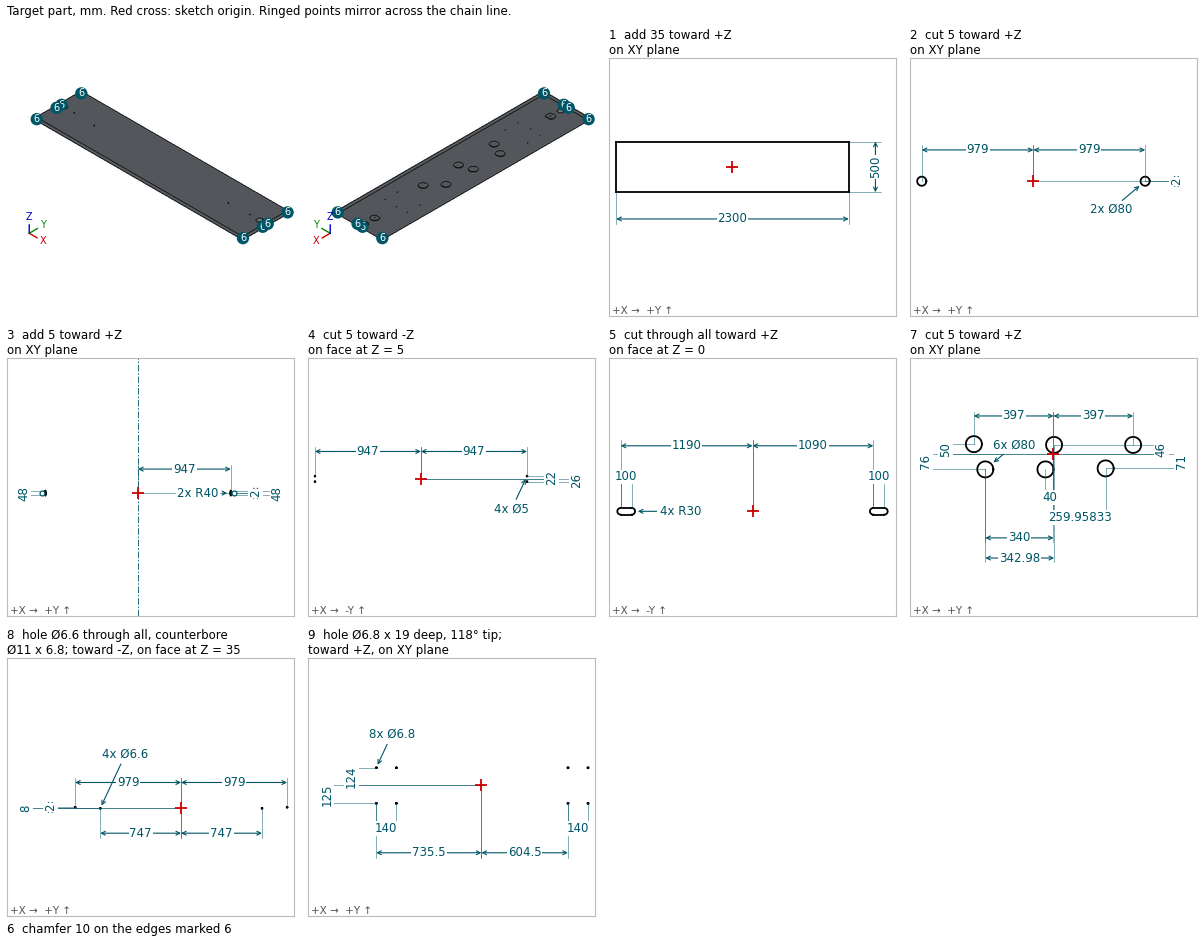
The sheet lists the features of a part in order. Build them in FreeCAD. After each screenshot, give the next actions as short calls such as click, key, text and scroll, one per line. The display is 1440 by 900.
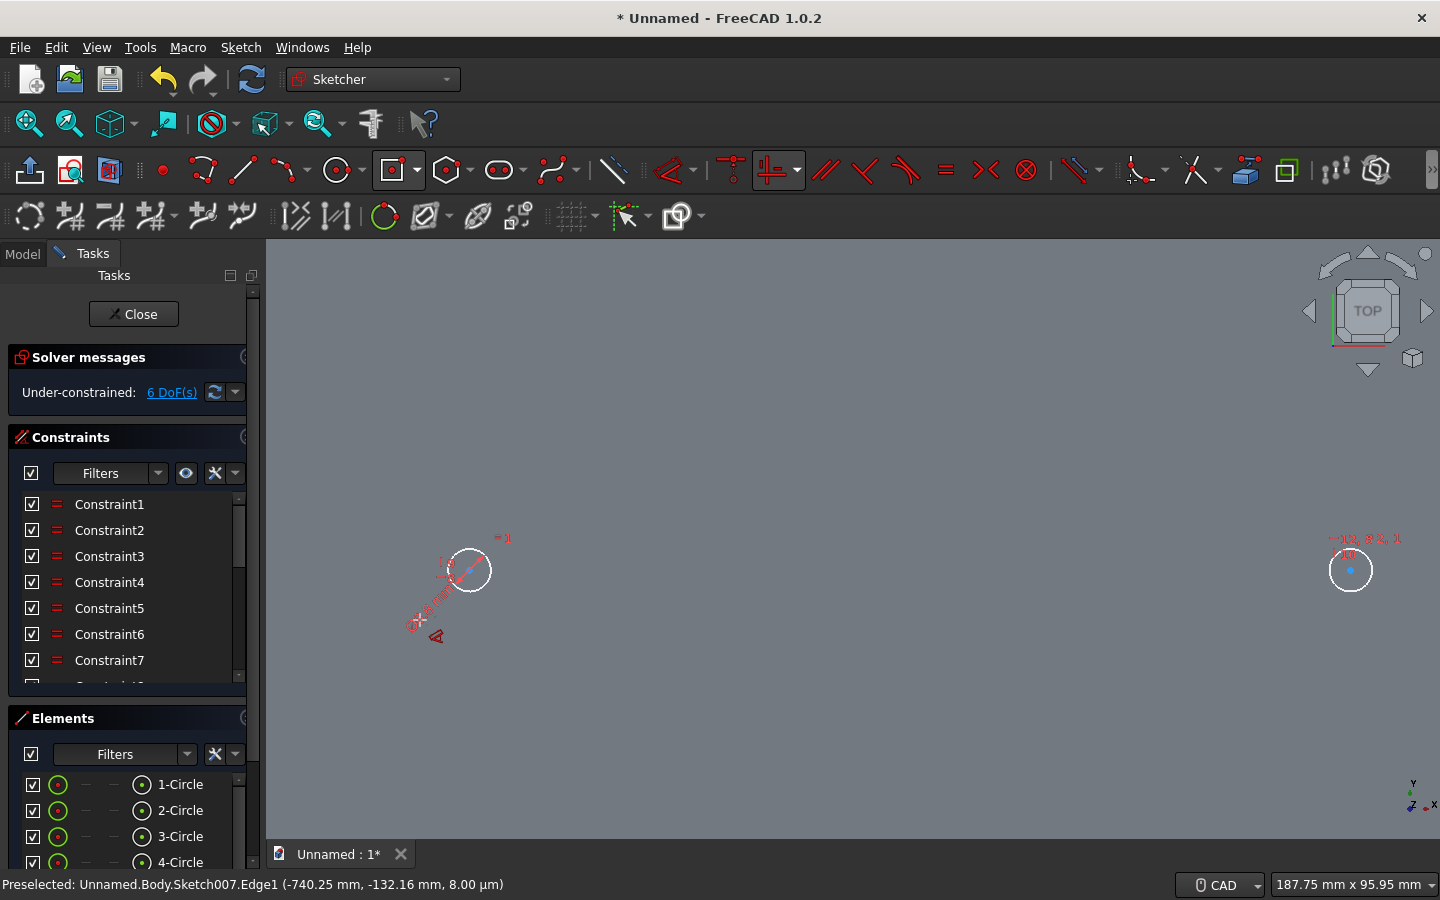
scroll(438, 600, down, 13)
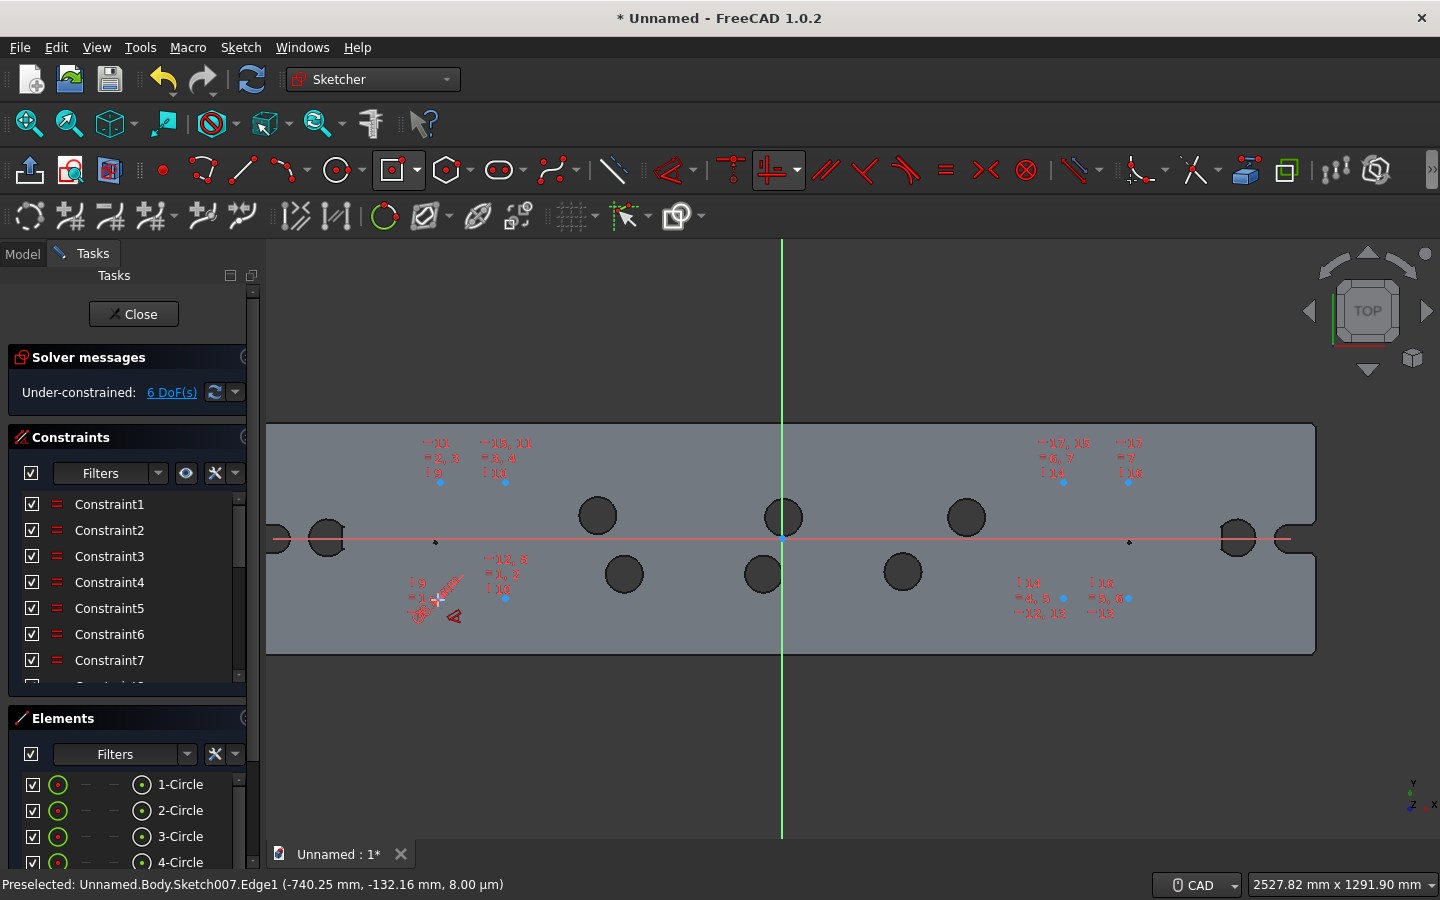
click(440, 598)
click(406, 569)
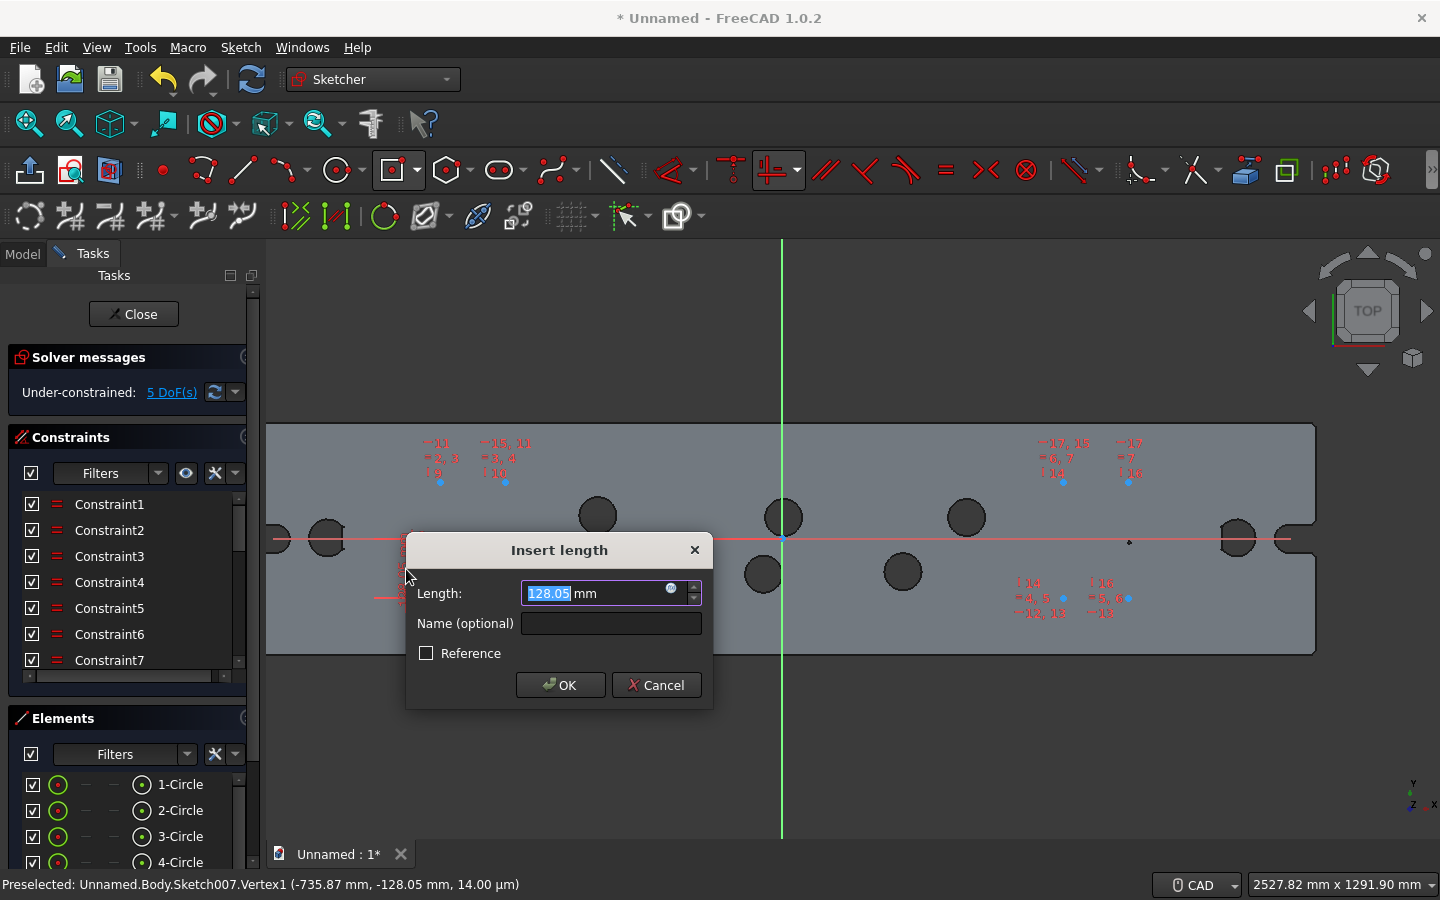
text(125)
key(Return)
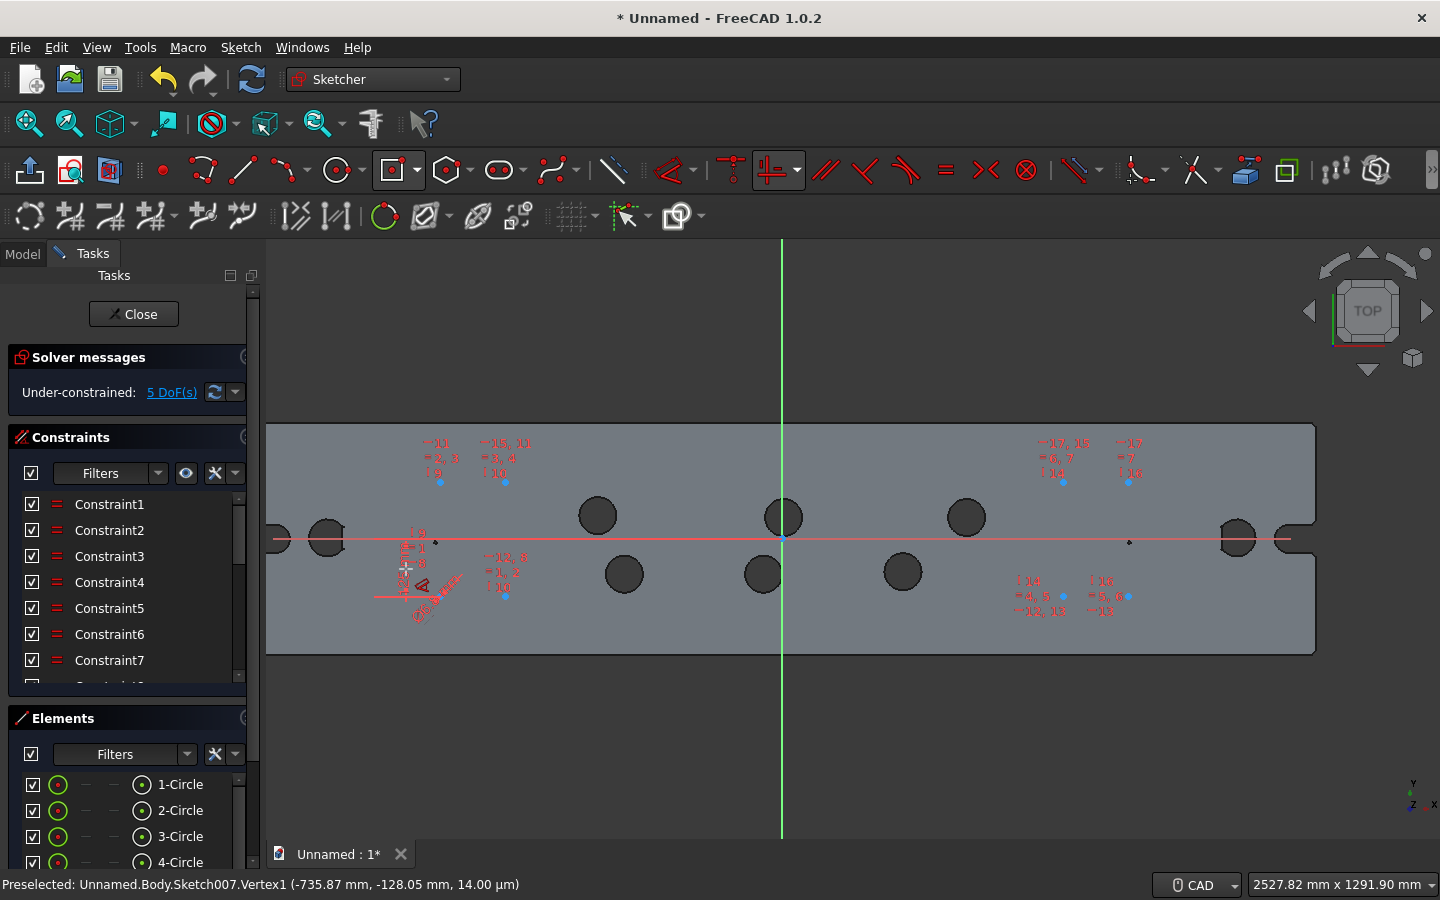
click(440, 483)
click(406, 511)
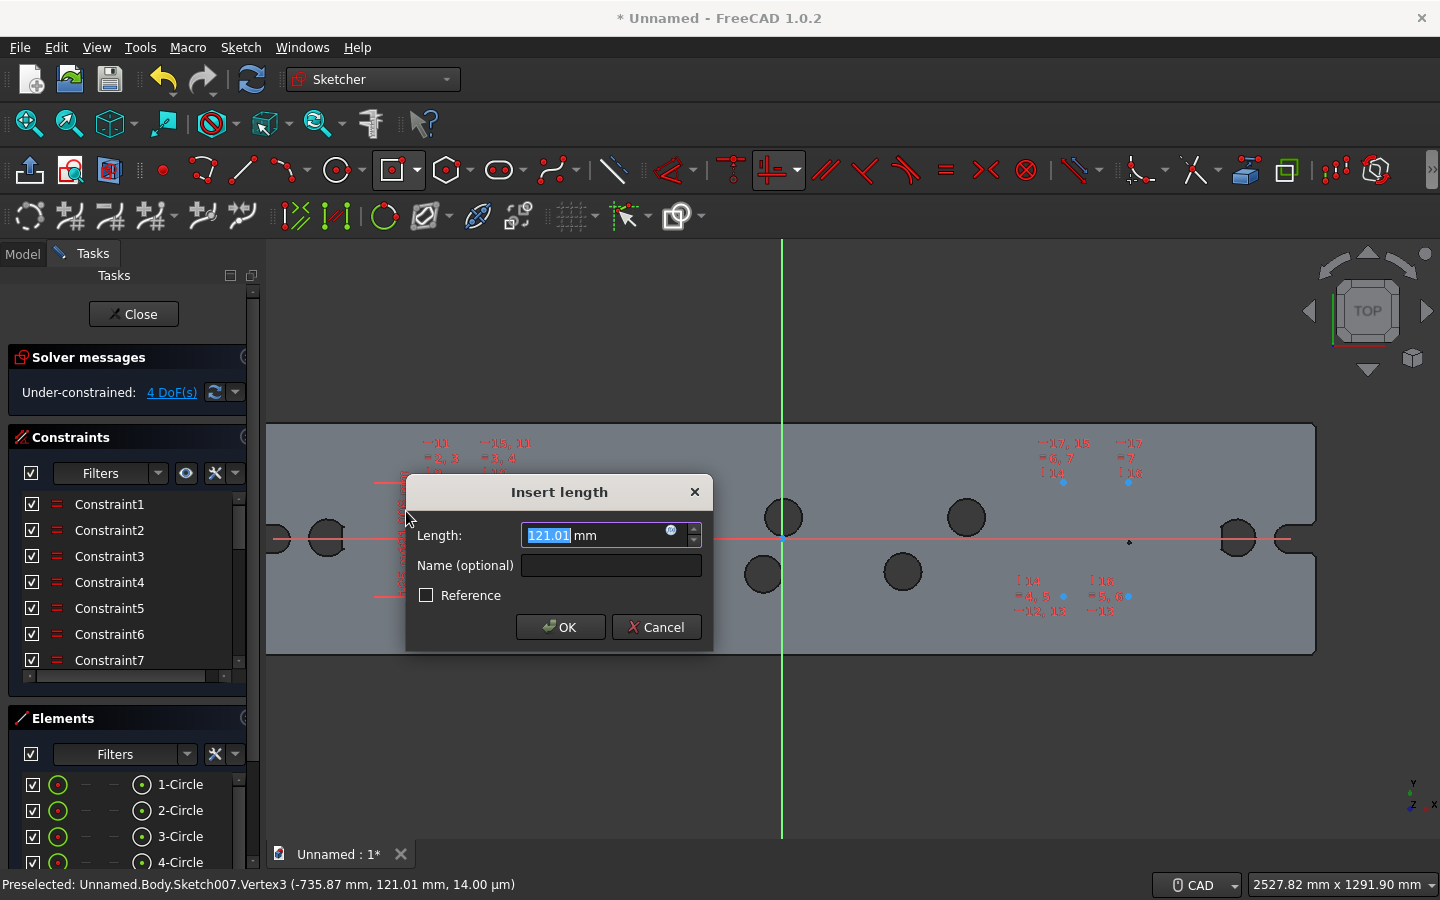
text(124)
key(Return)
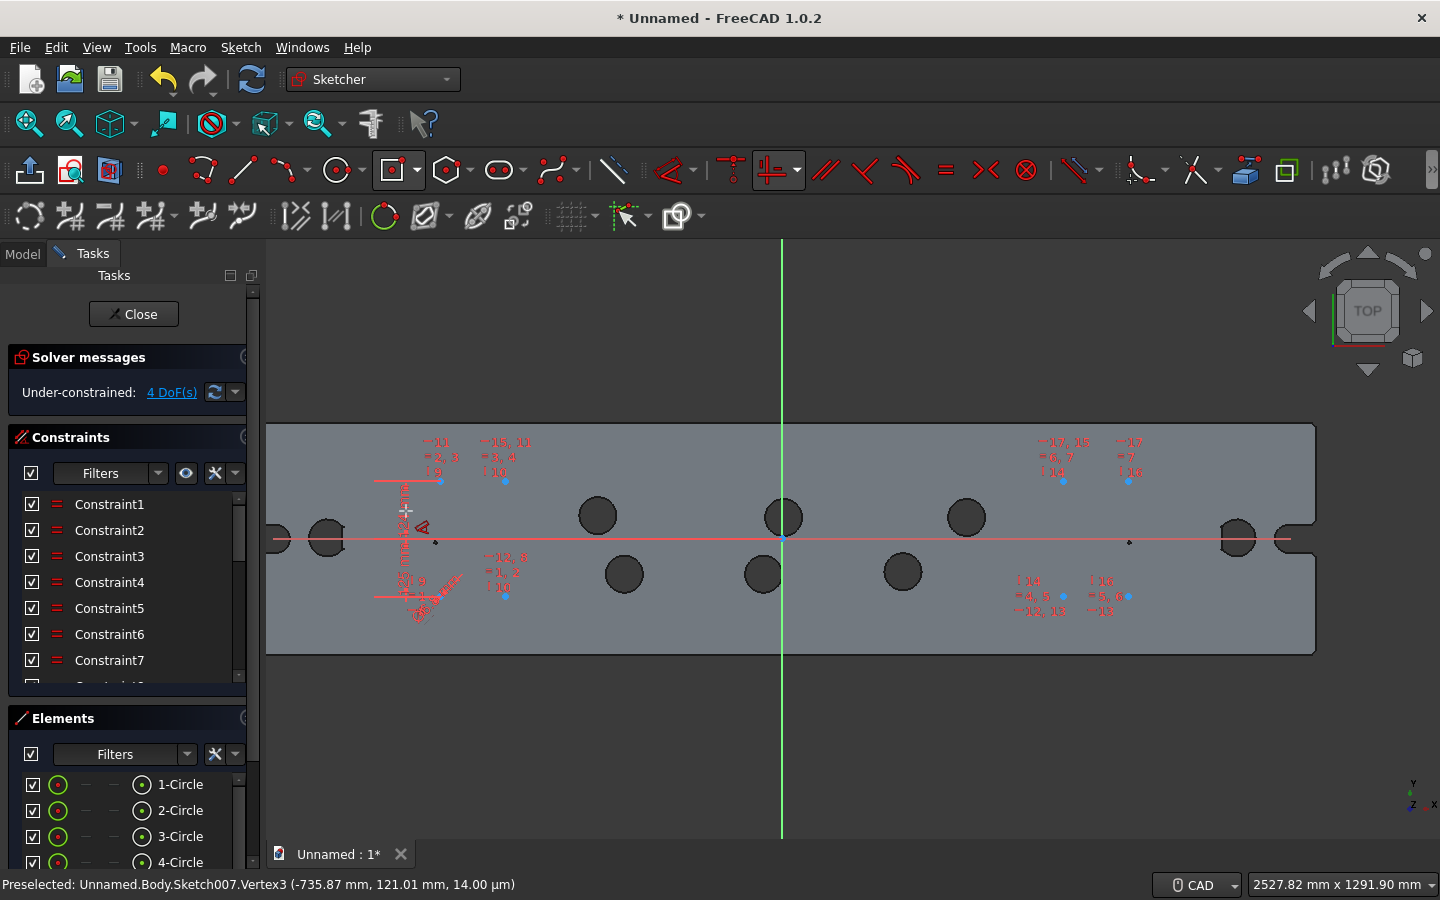
click(440, 597)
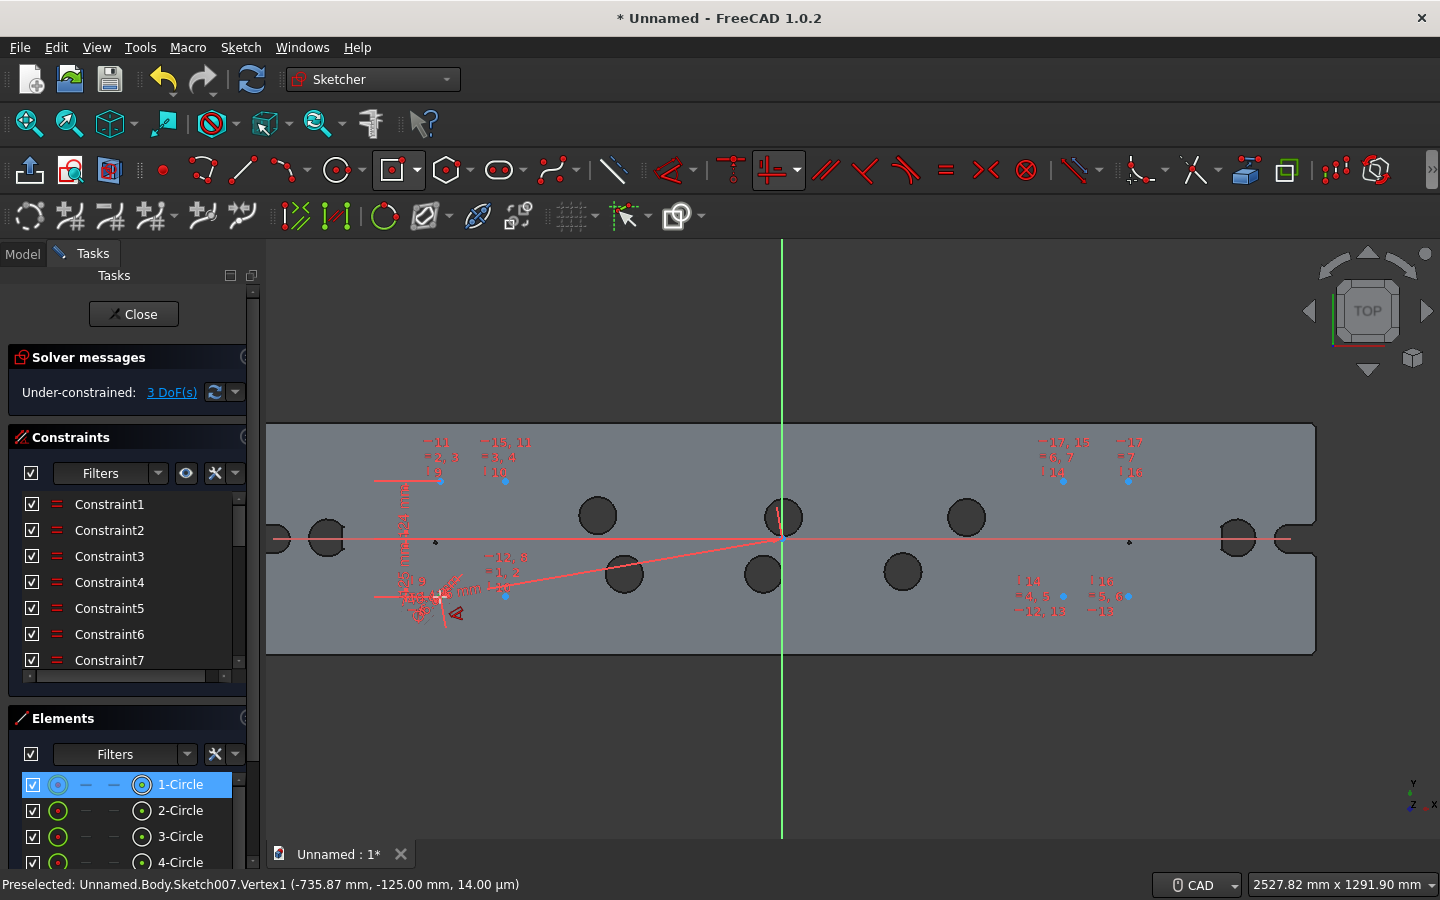
click(506, 597)
click(473, 631)